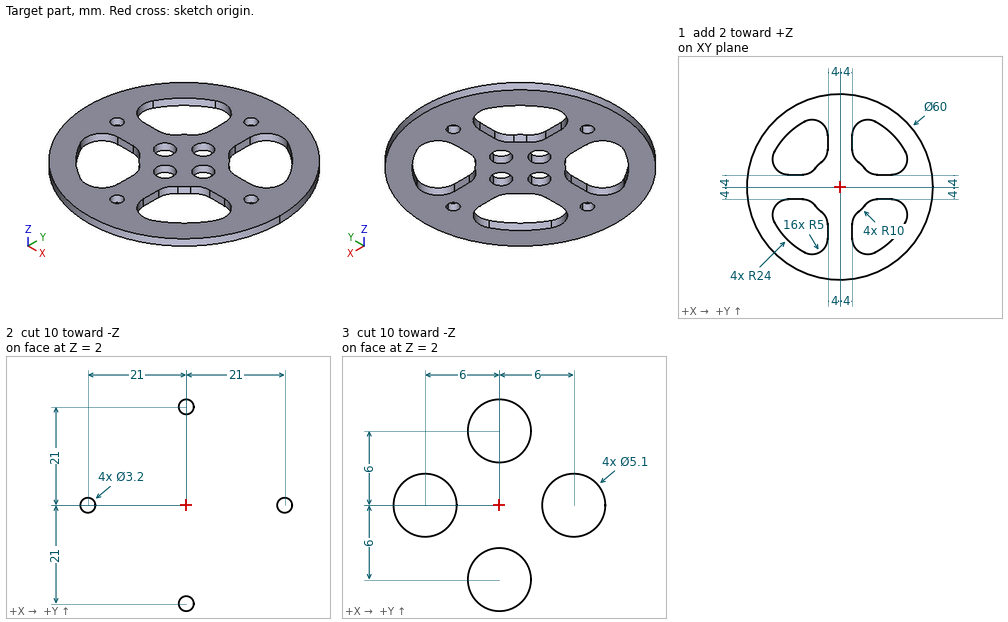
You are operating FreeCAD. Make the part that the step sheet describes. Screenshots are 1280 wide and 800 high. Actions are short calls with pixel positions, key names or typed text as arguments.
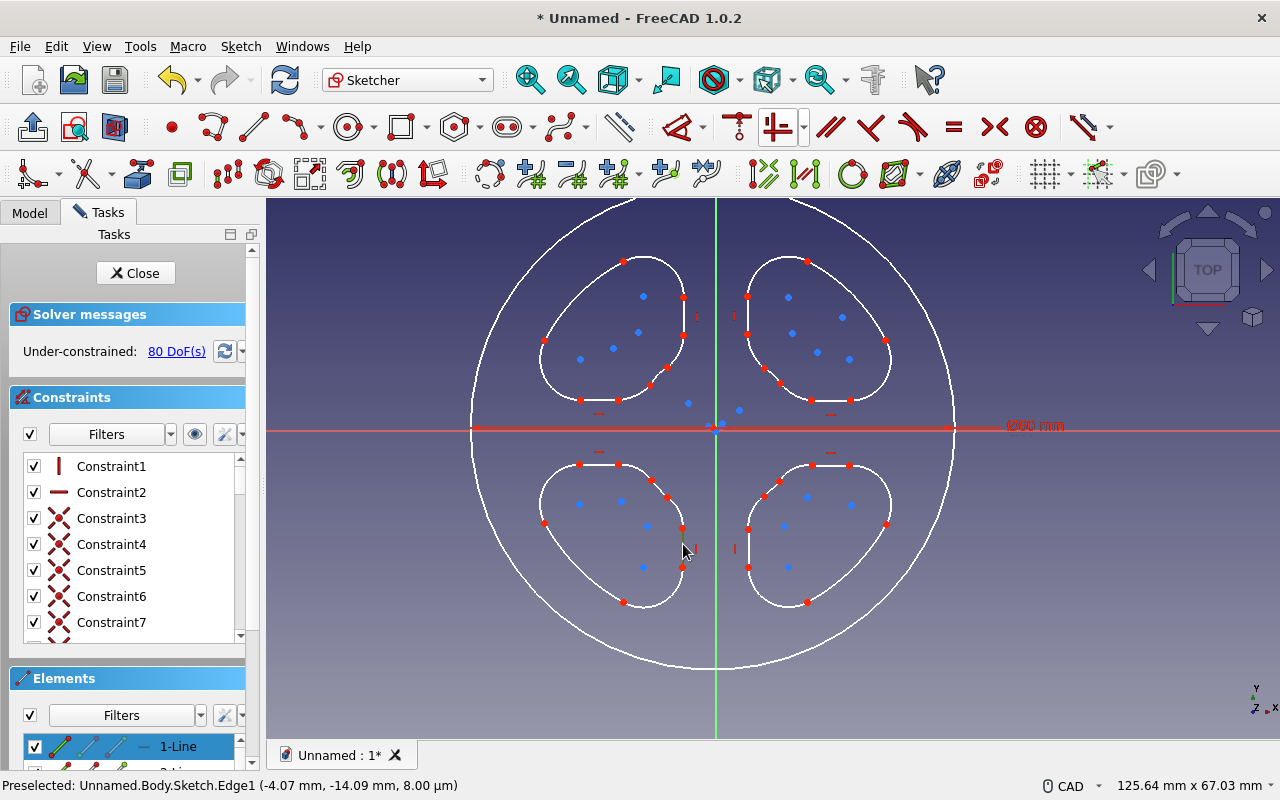
click(648, 607)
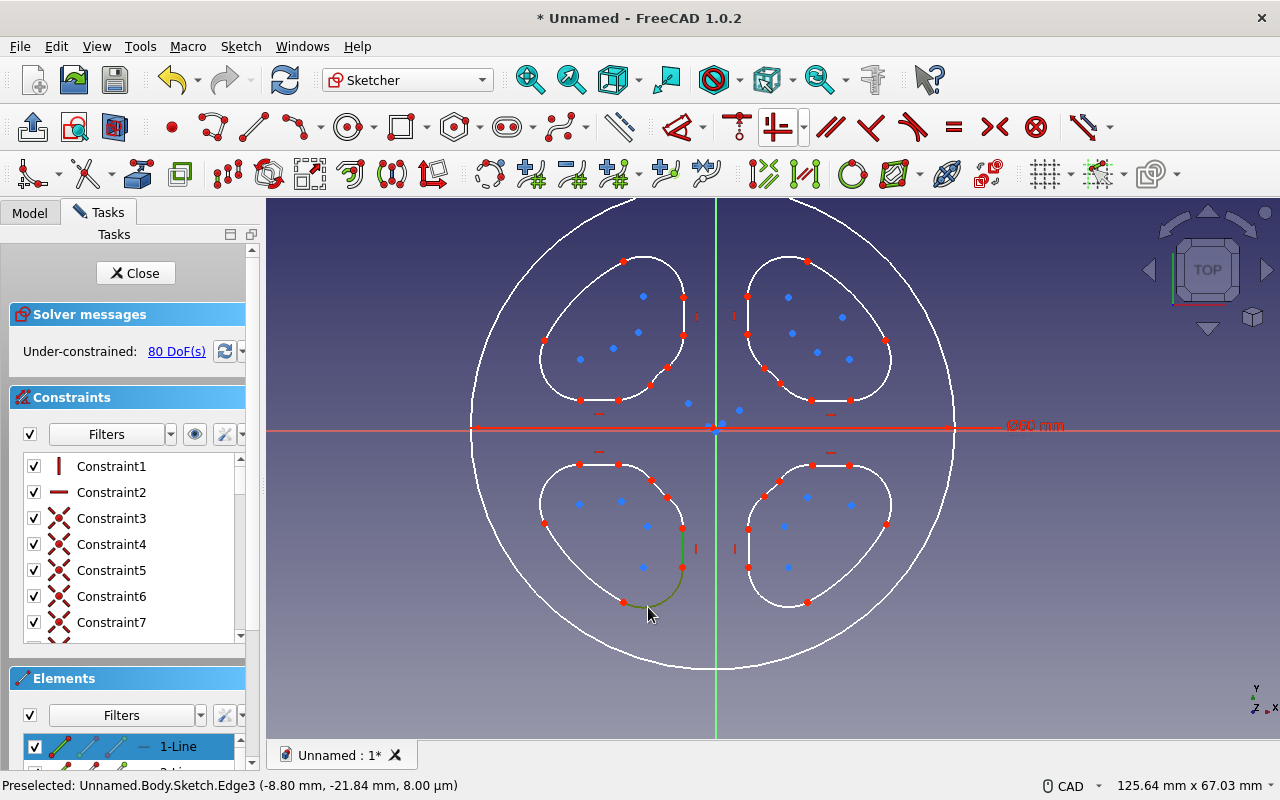
key(t)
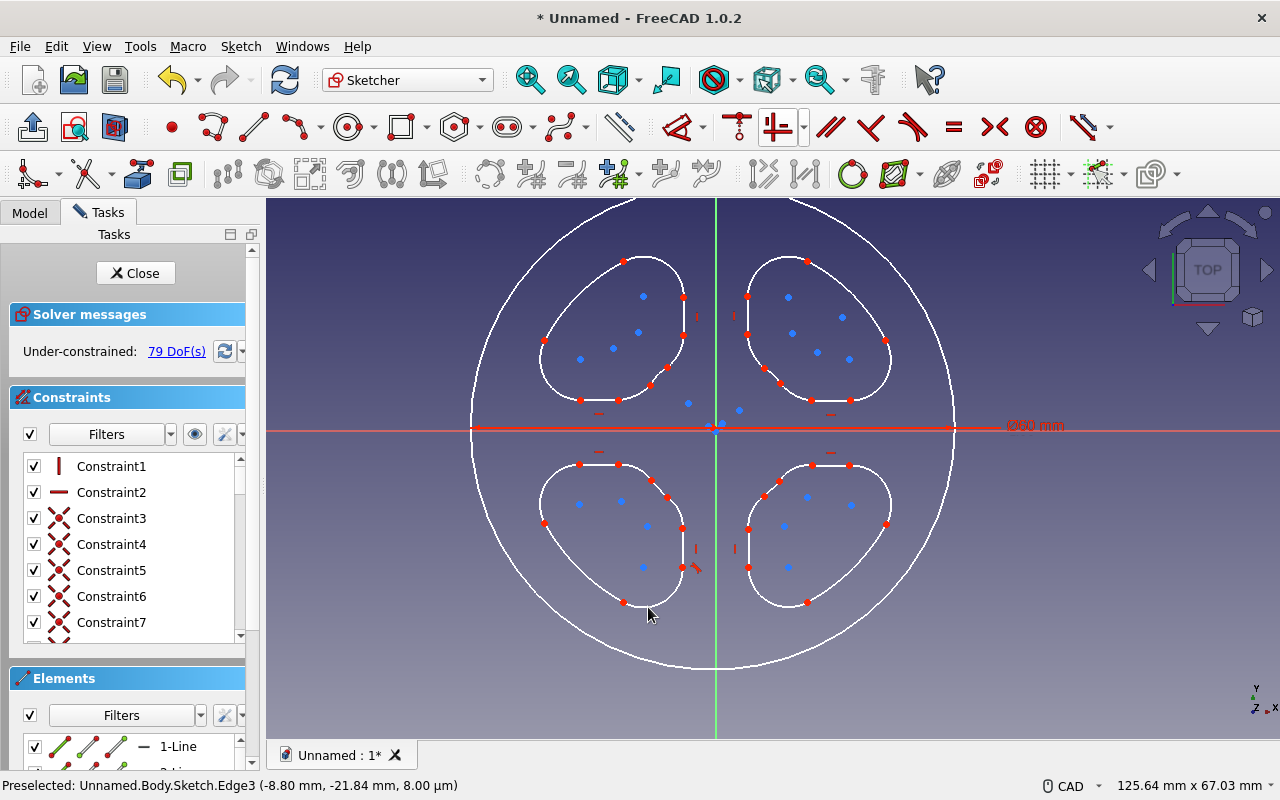
click(683, 541)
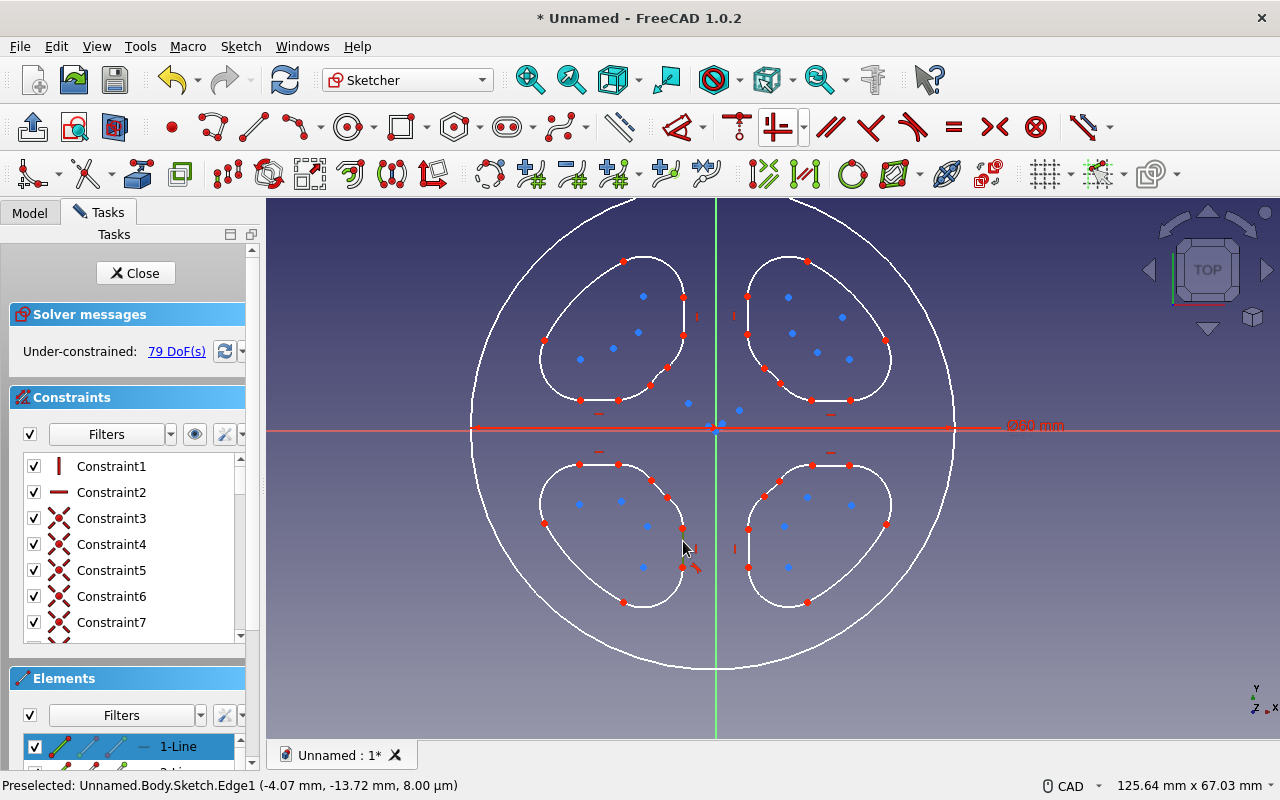
scroll(682, 518, up, 2)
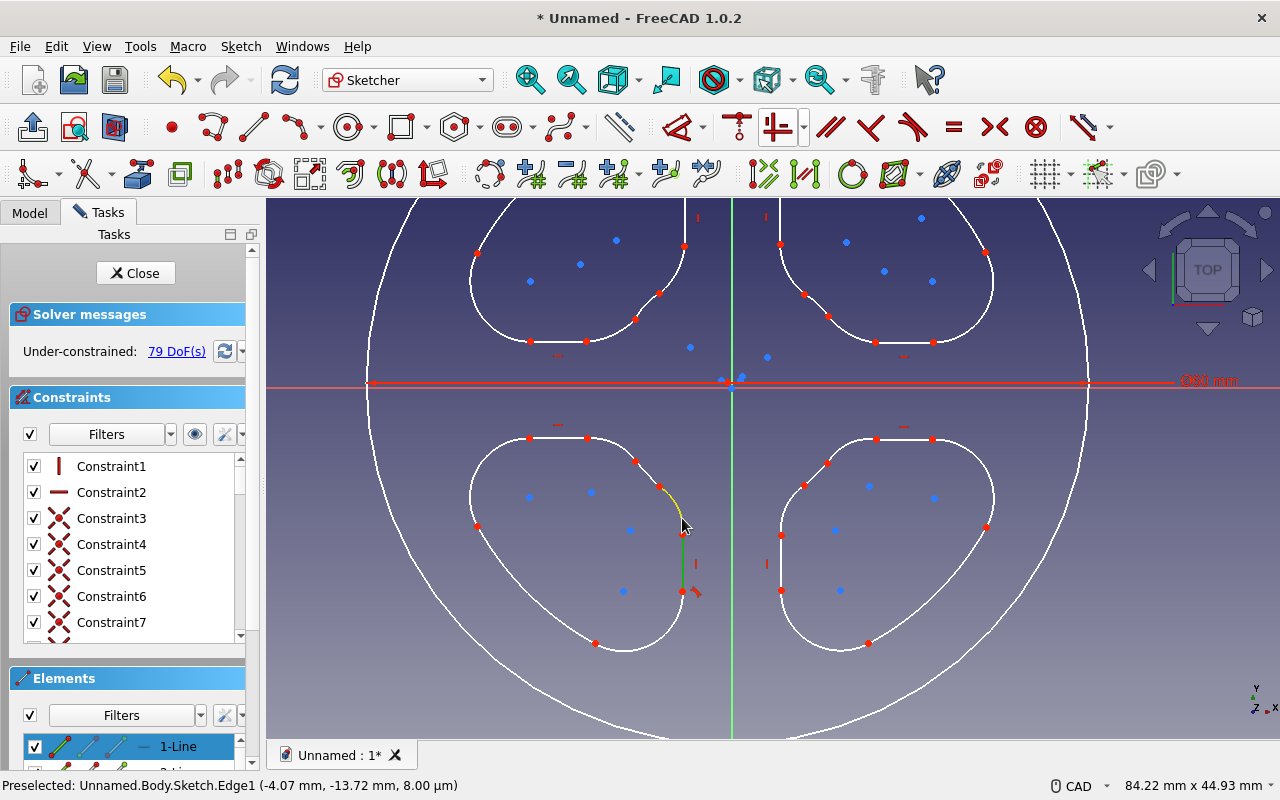
click(681, 518)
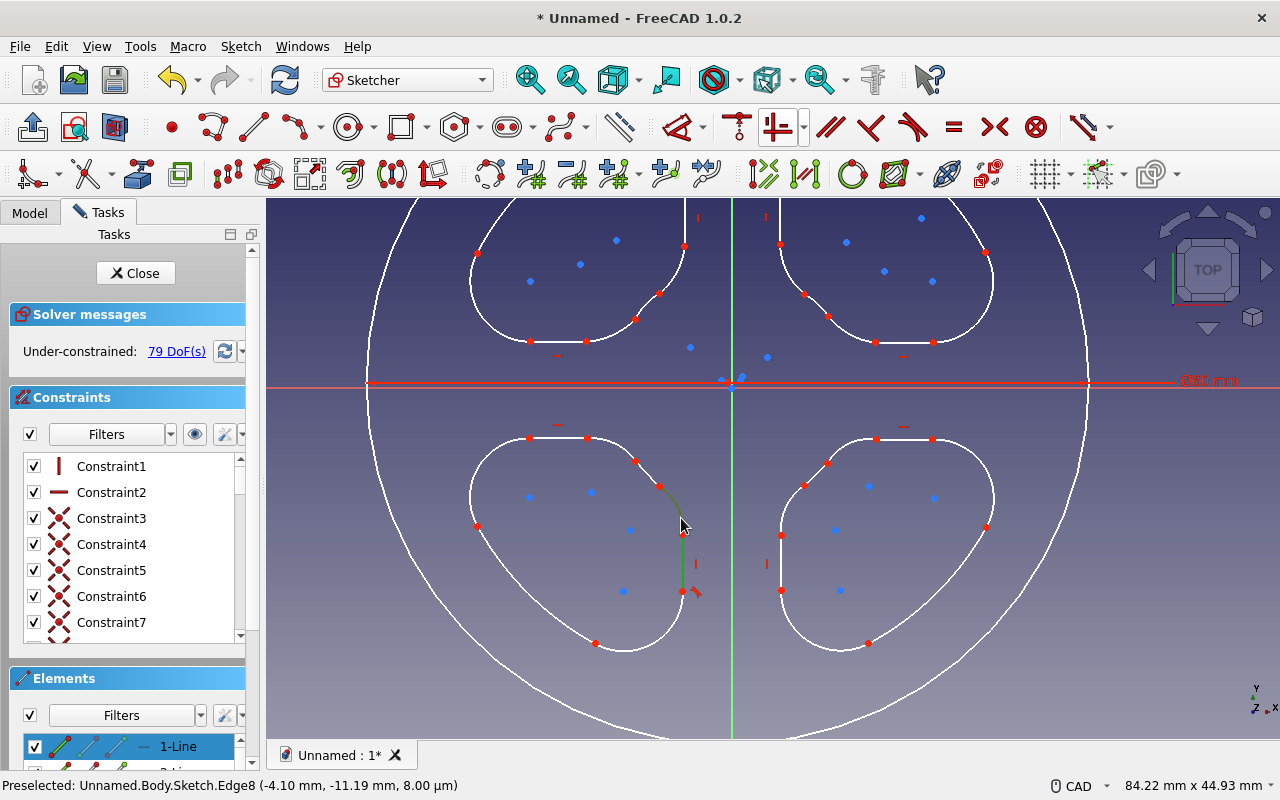
click(913, 128)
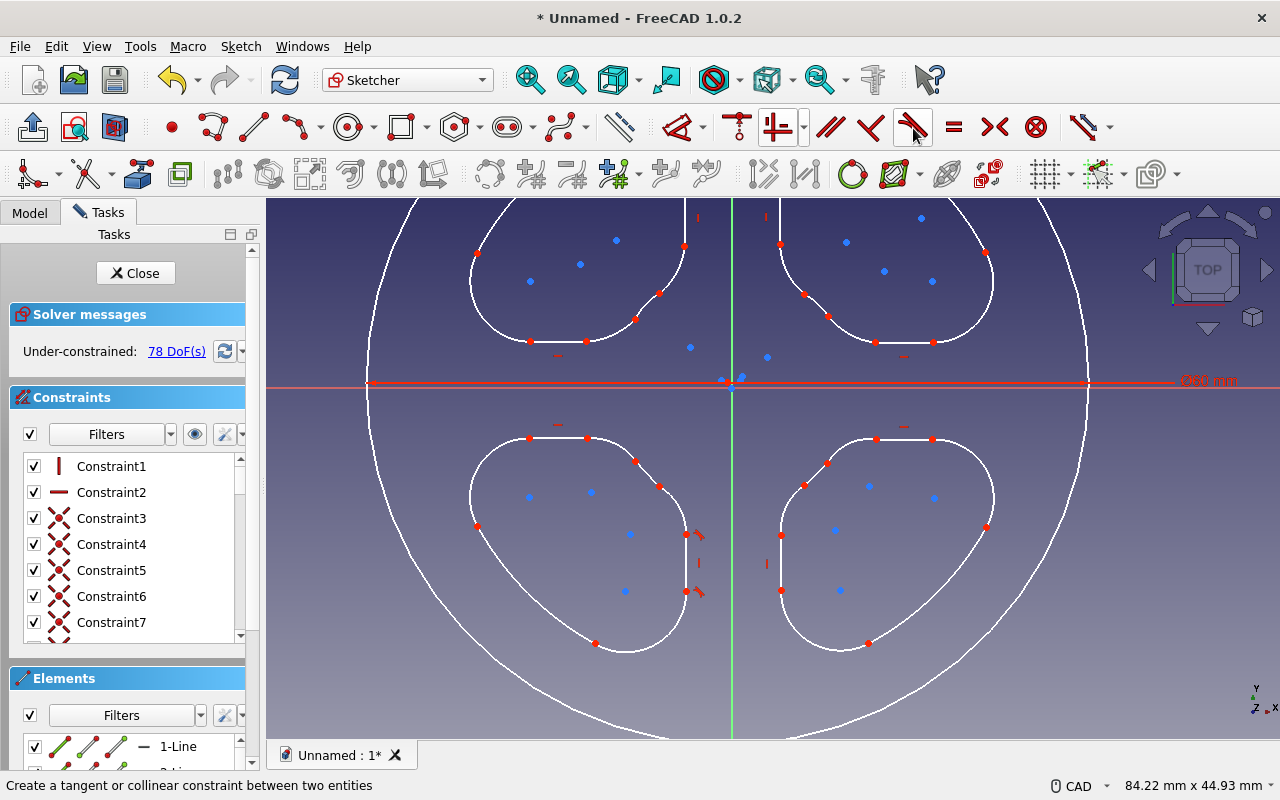
click(547, 438)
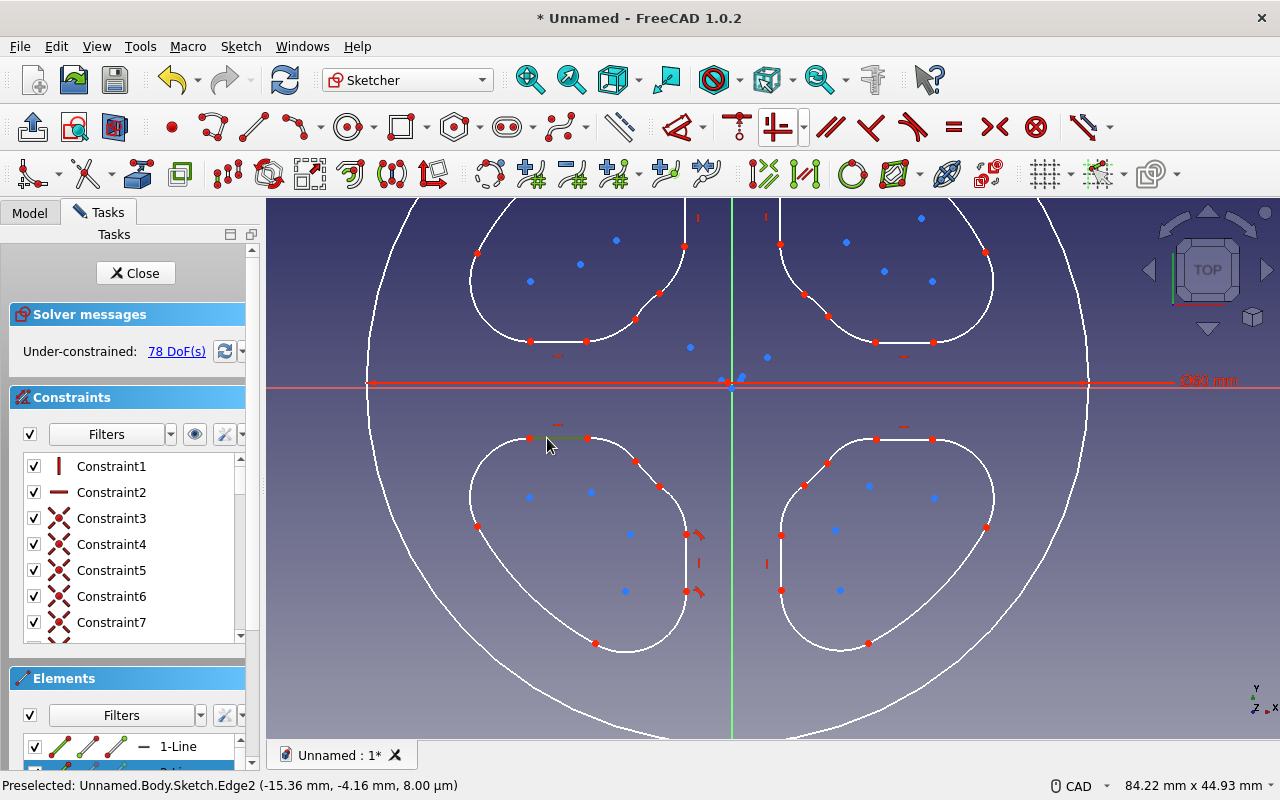
click(495, 449)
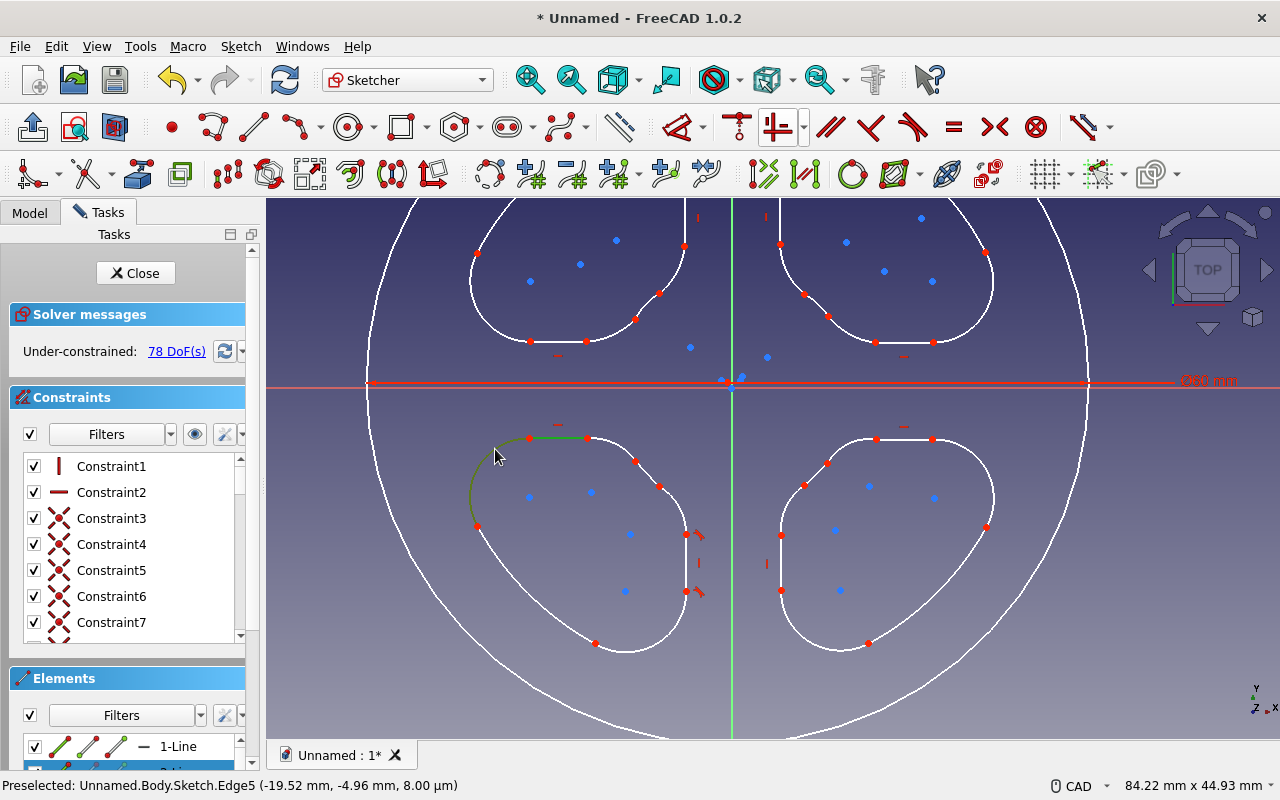
click(913, 128)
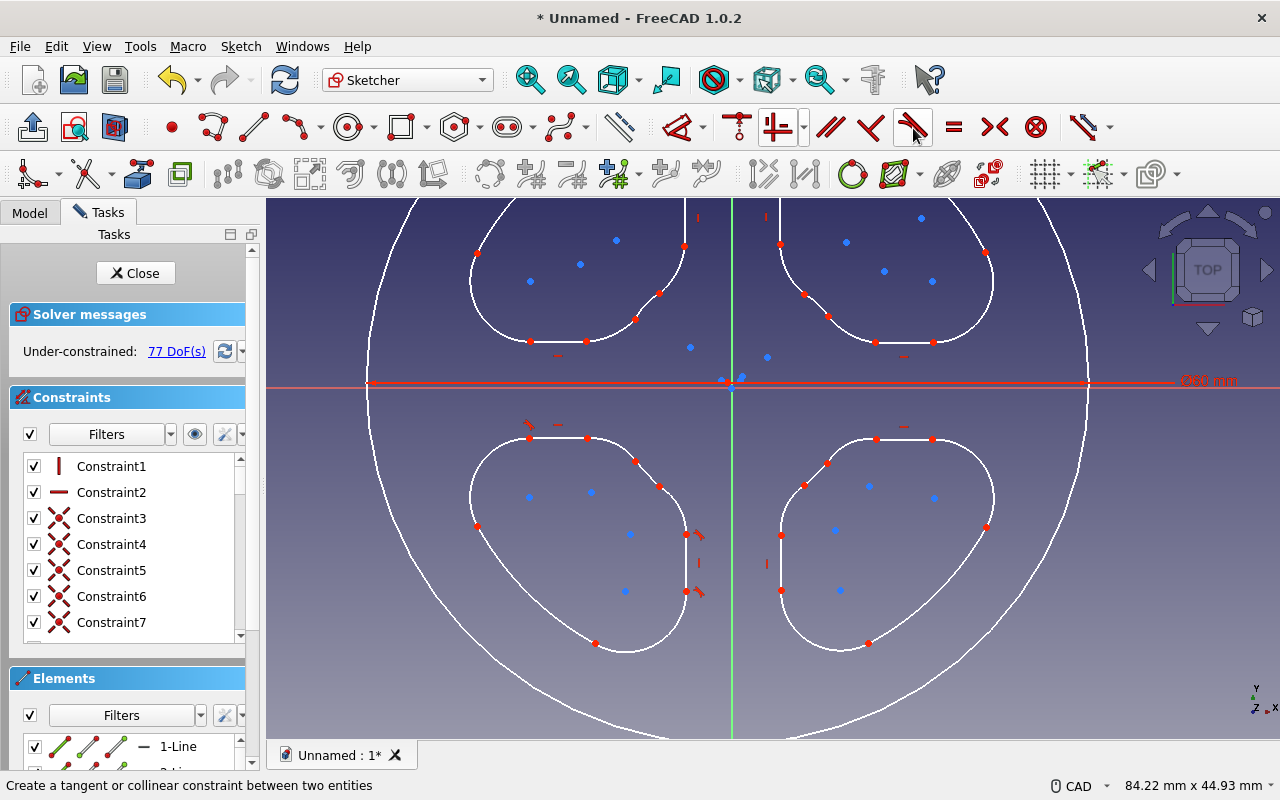
click(547, 438)